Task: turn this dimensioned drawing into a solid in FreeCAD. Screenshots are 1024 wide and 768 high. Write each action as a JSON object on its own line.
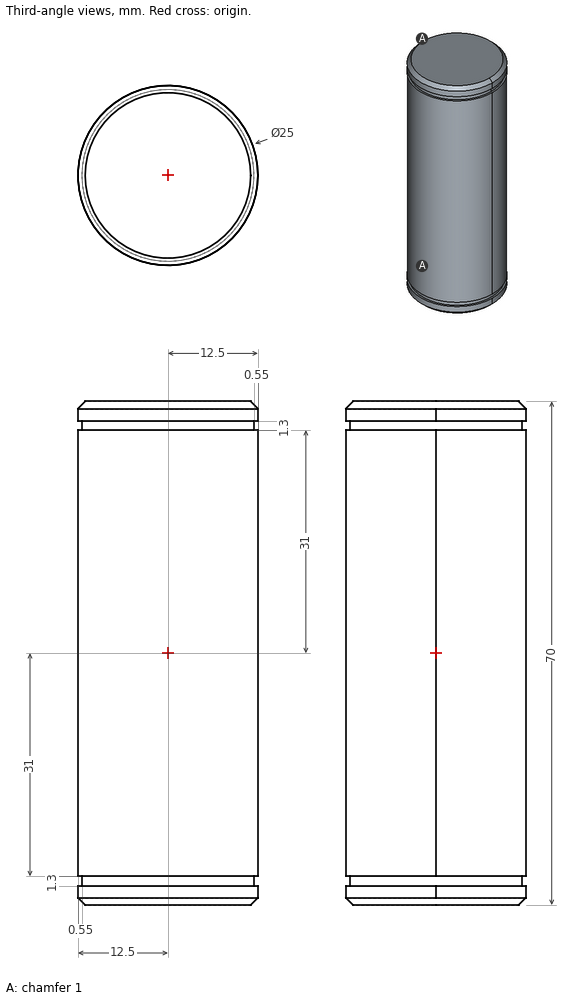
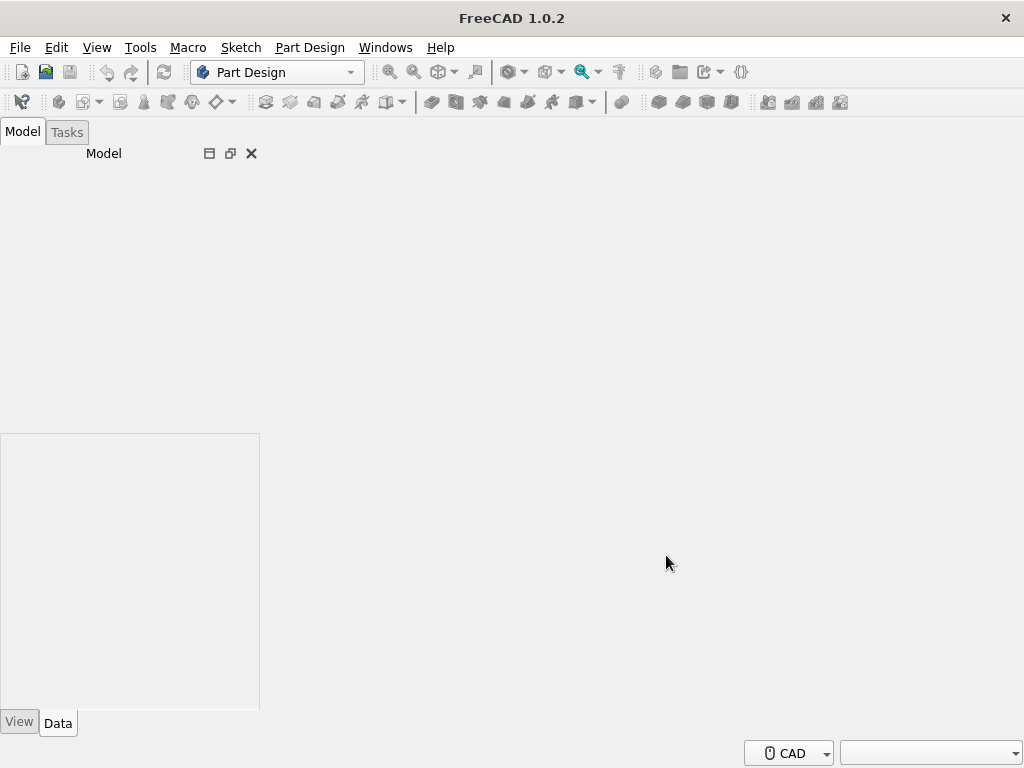
{"action": "left_click", "coordinate": [22, 72]}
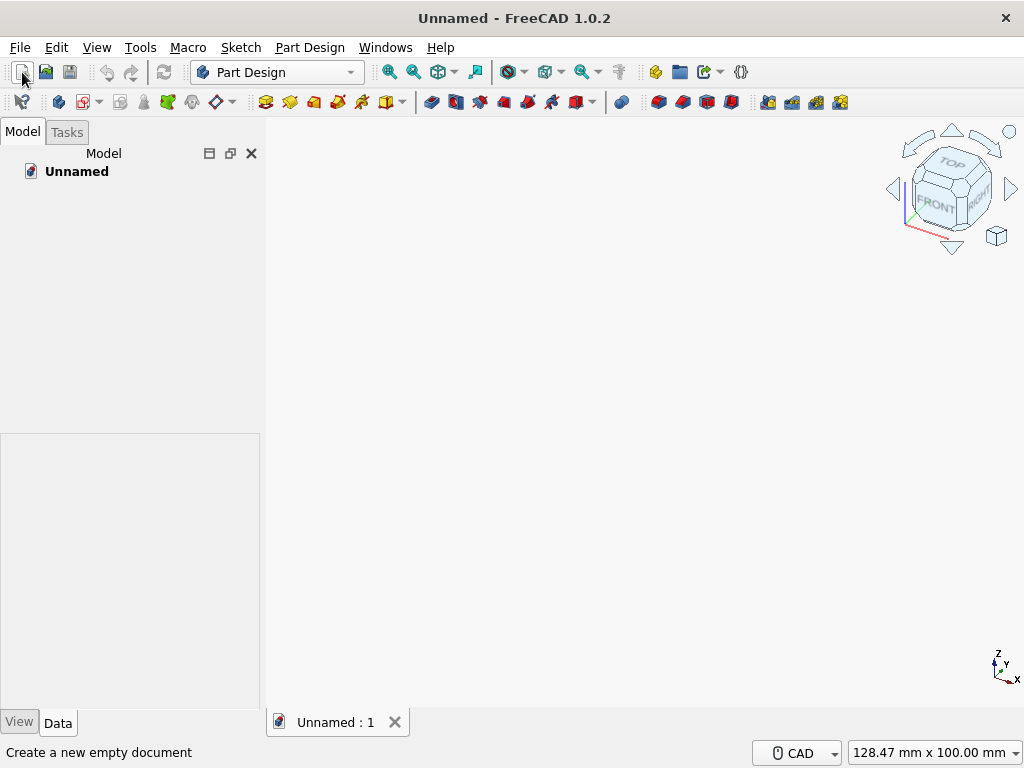
{"action": "left_click", "coordinate": [84, 102]}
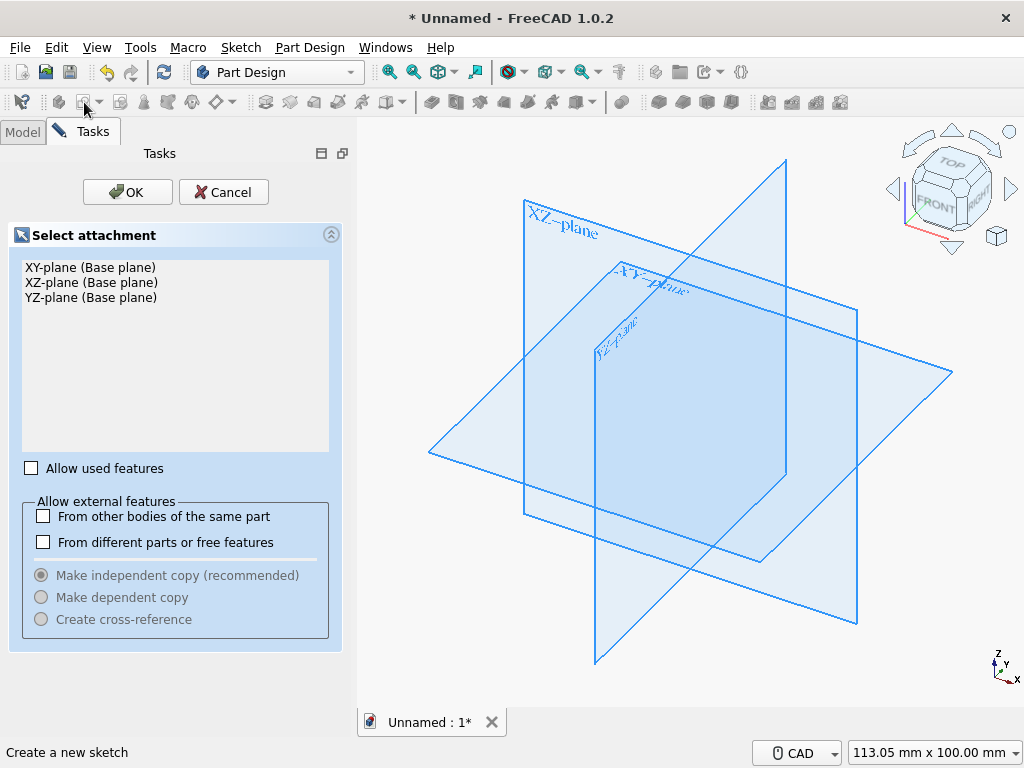
{"action": "left_click", "coordinate": [82, 268]}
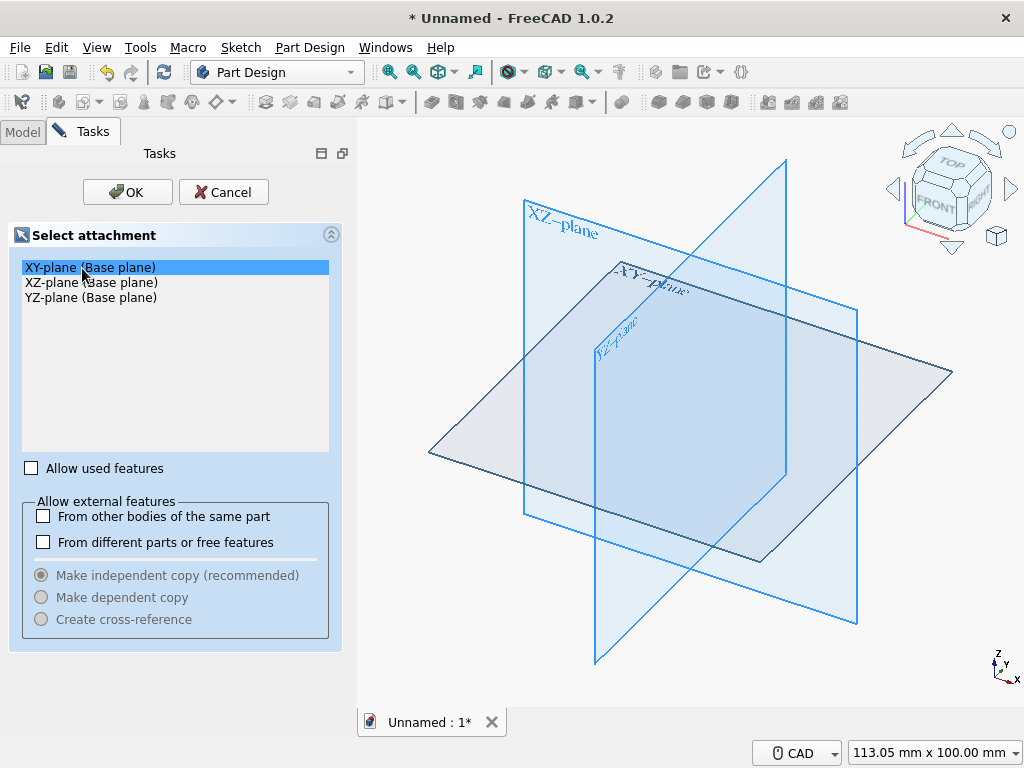
{"action": "left_click", "coordinate": [128, 192]}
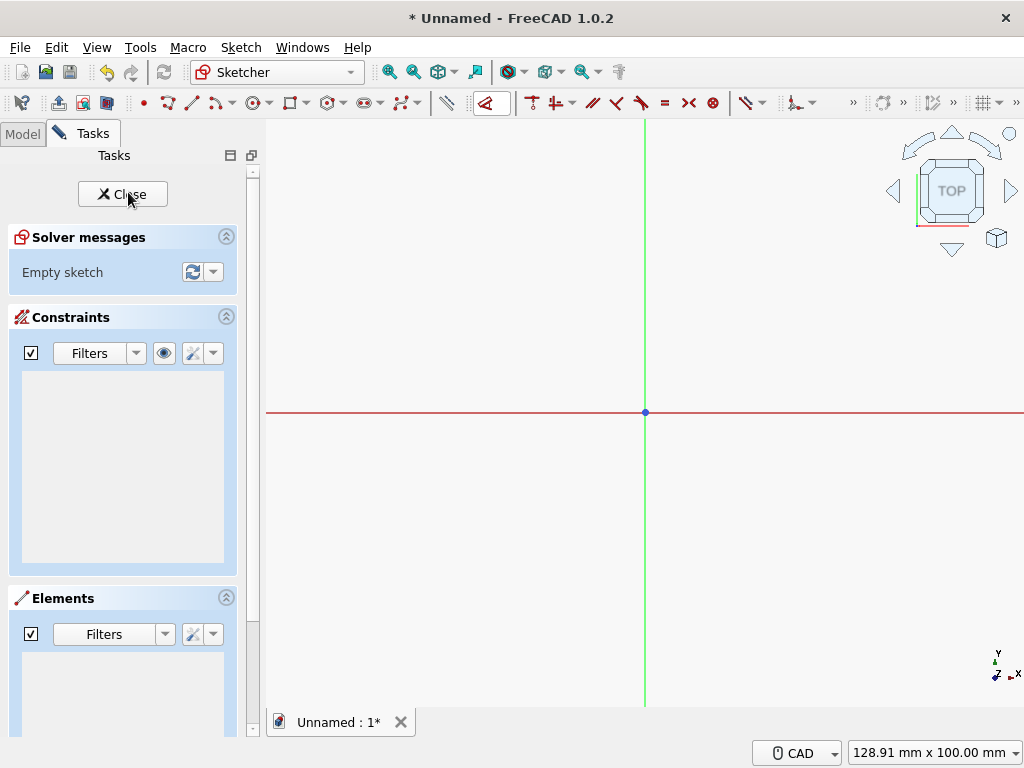
{"action": "scroll", "coordinate": [685, 413], "scroll_direction": "up", "scroll_amount": 5}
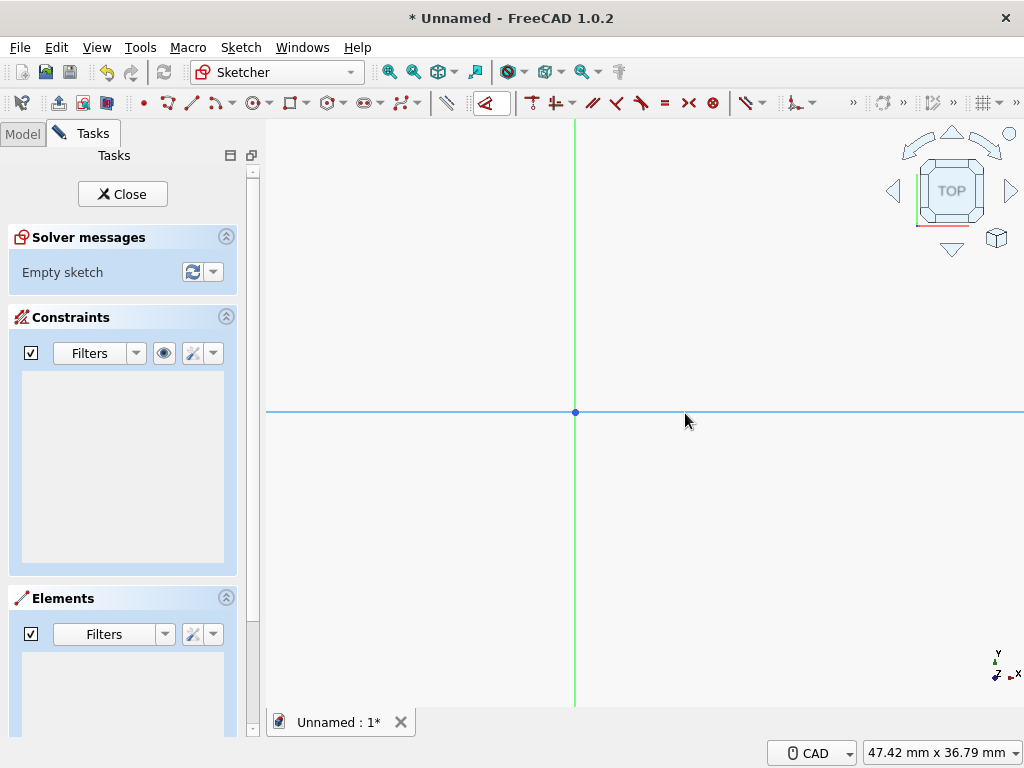
{"action": "key", "text": "g c"}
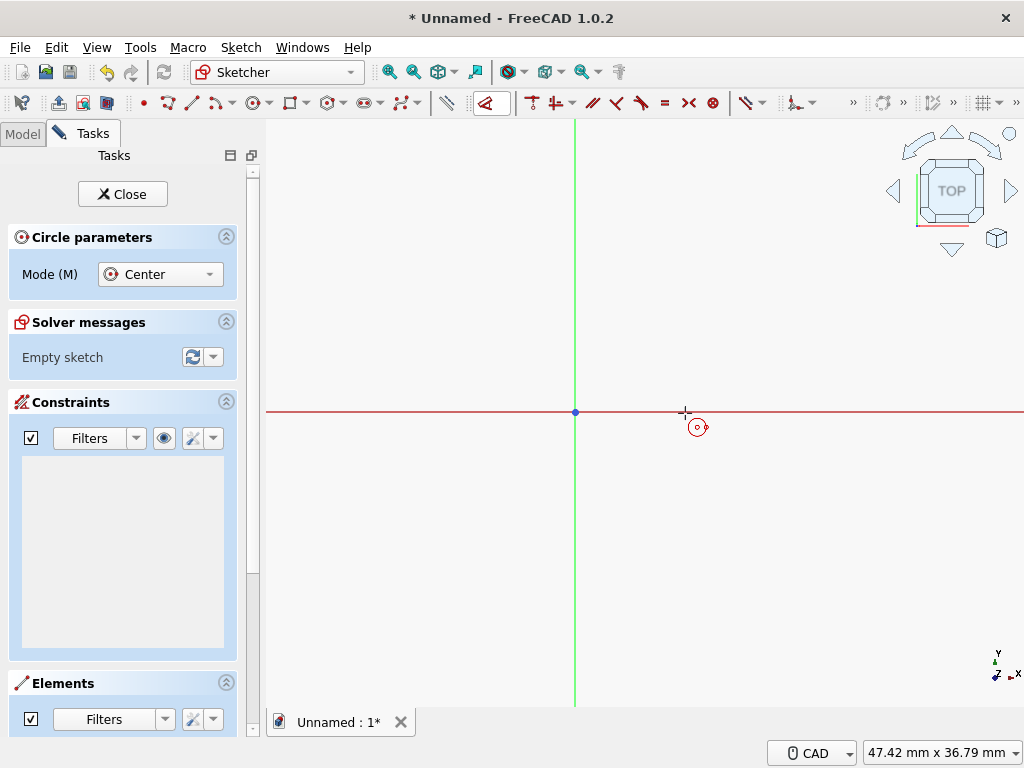
{"action": "left_click", "coordinate": [575, 412]}
{"action": "left_click", "coordinate": [717, 271]}
{"action": "key", "text": "Escape"}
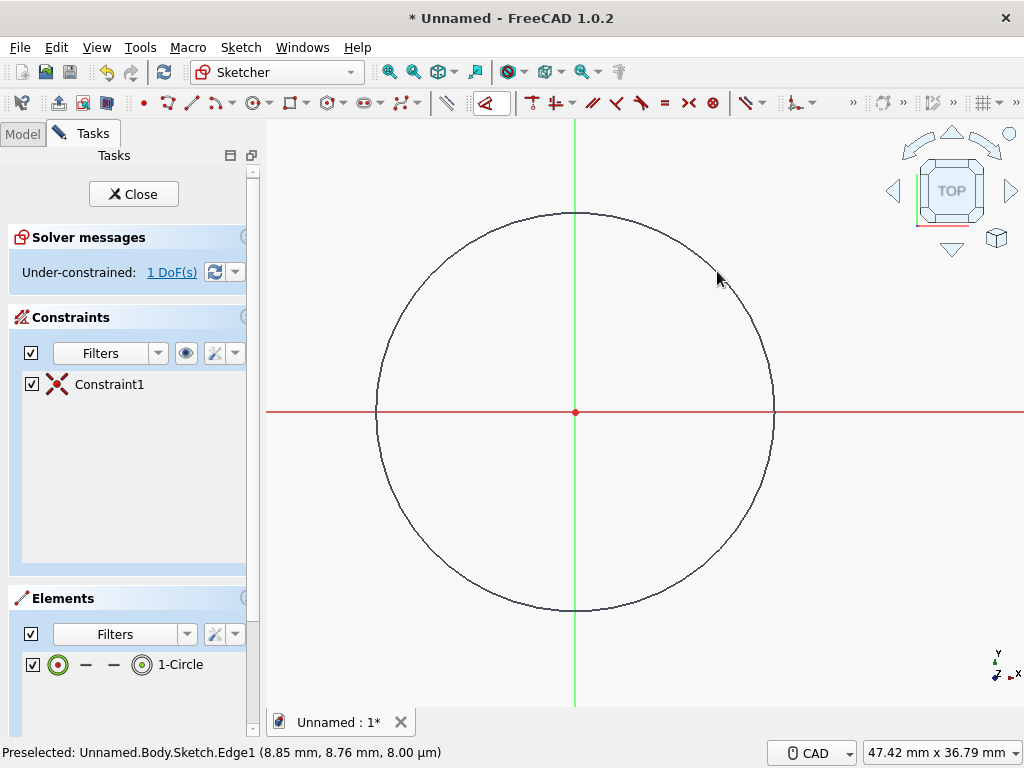
{"action": "key", "text": "d"}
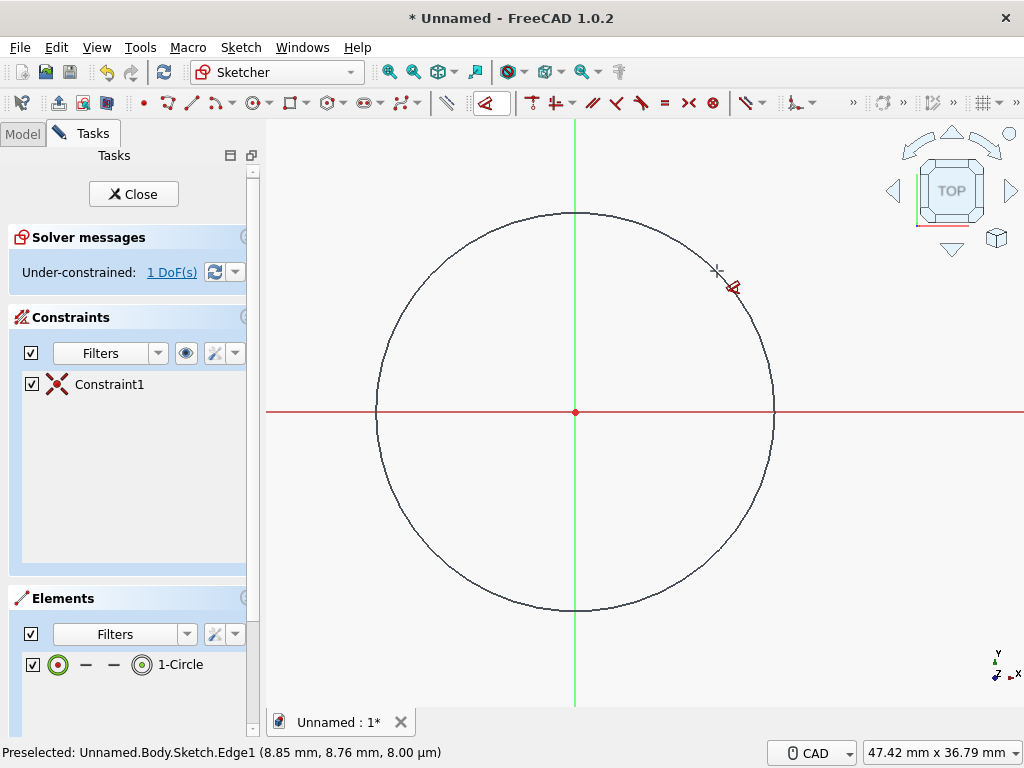
{"action": "left_click", "coordinate": [716, 271]}
{"action": "left_click", "coordinate": [739, 248]}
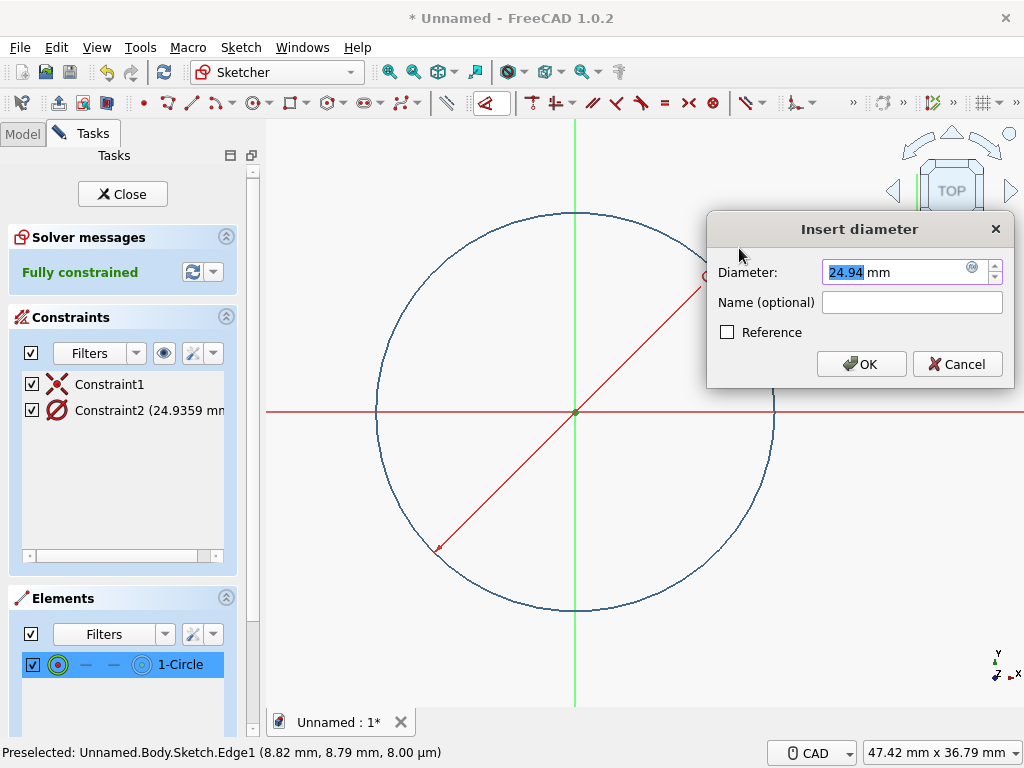
{"action": "type", "text": "25"}
{"action": "key", "text": "Return"}
{"action": "key", "text": "Escape"}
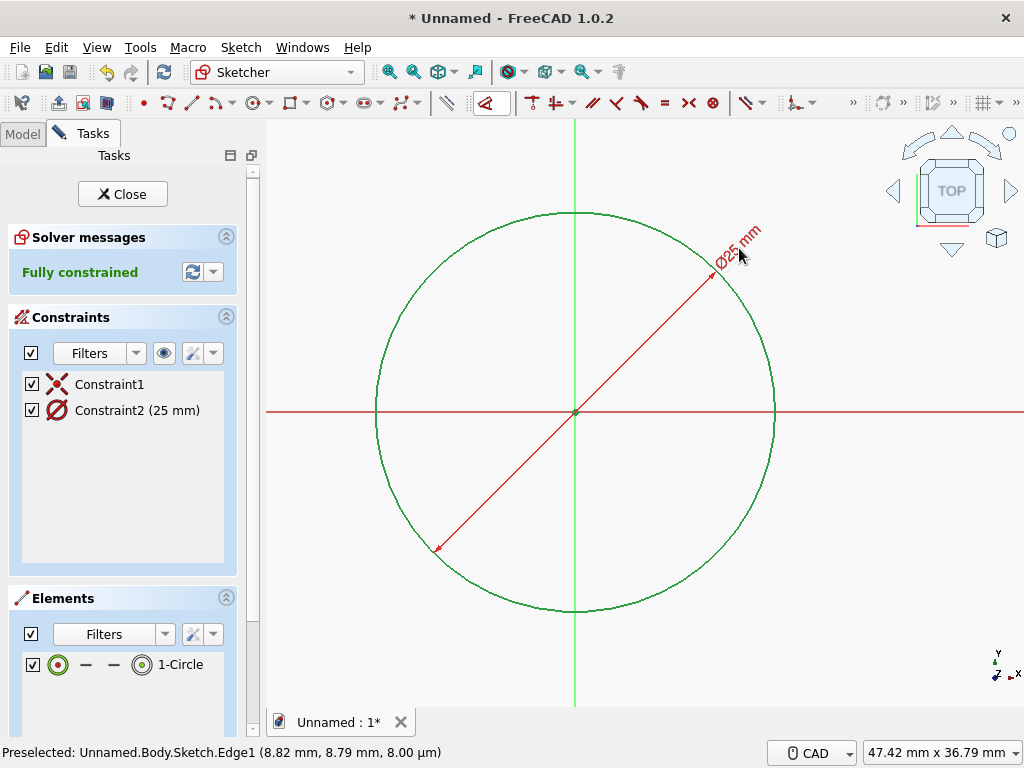
{"action": "left_click", "coordinate": [123, 194]}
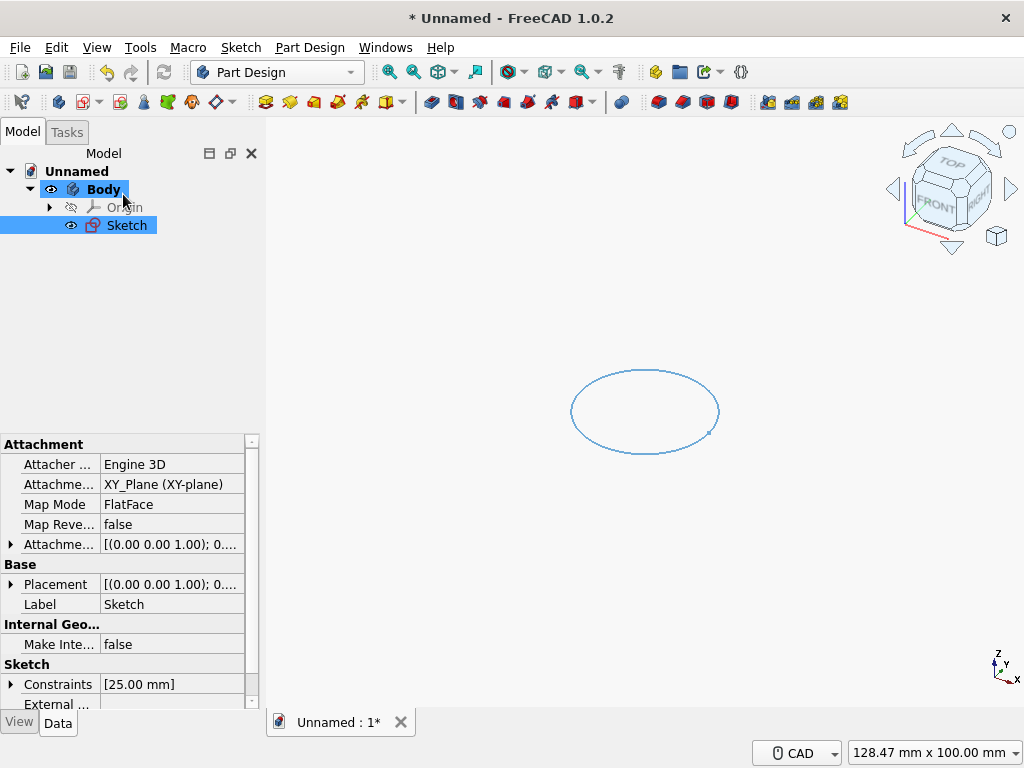
{"action": "left_click", "coordinate": [266, 102]}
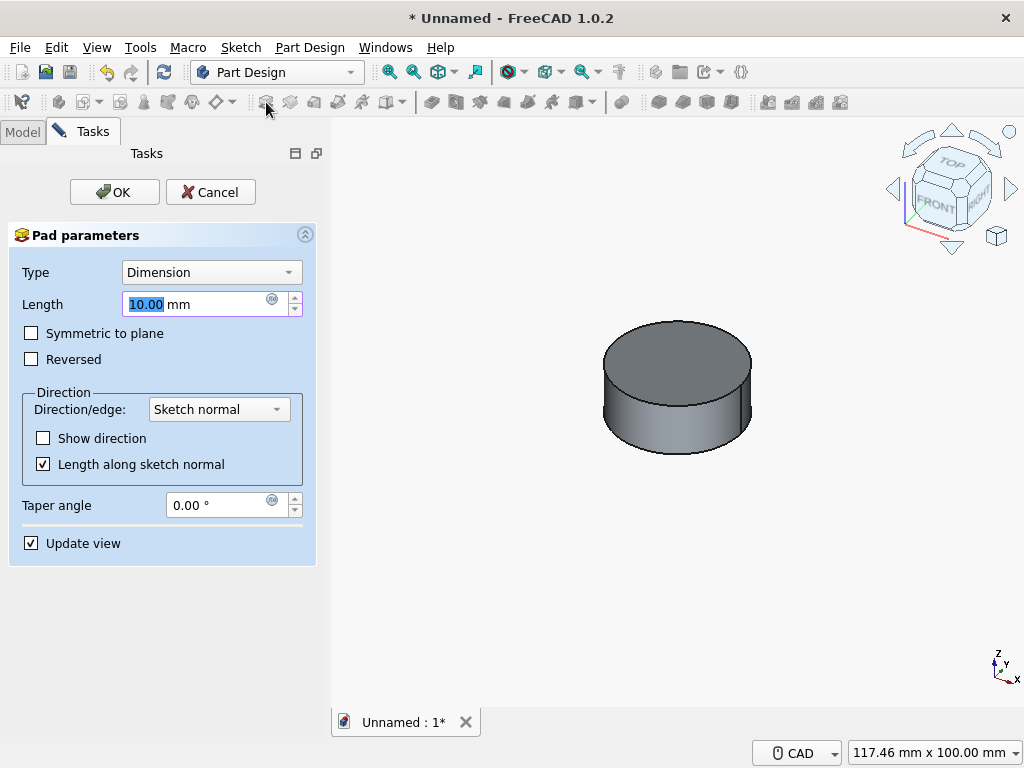
{"action": "type", "text": "70"}
{"action": "key", "text": "Tab"}